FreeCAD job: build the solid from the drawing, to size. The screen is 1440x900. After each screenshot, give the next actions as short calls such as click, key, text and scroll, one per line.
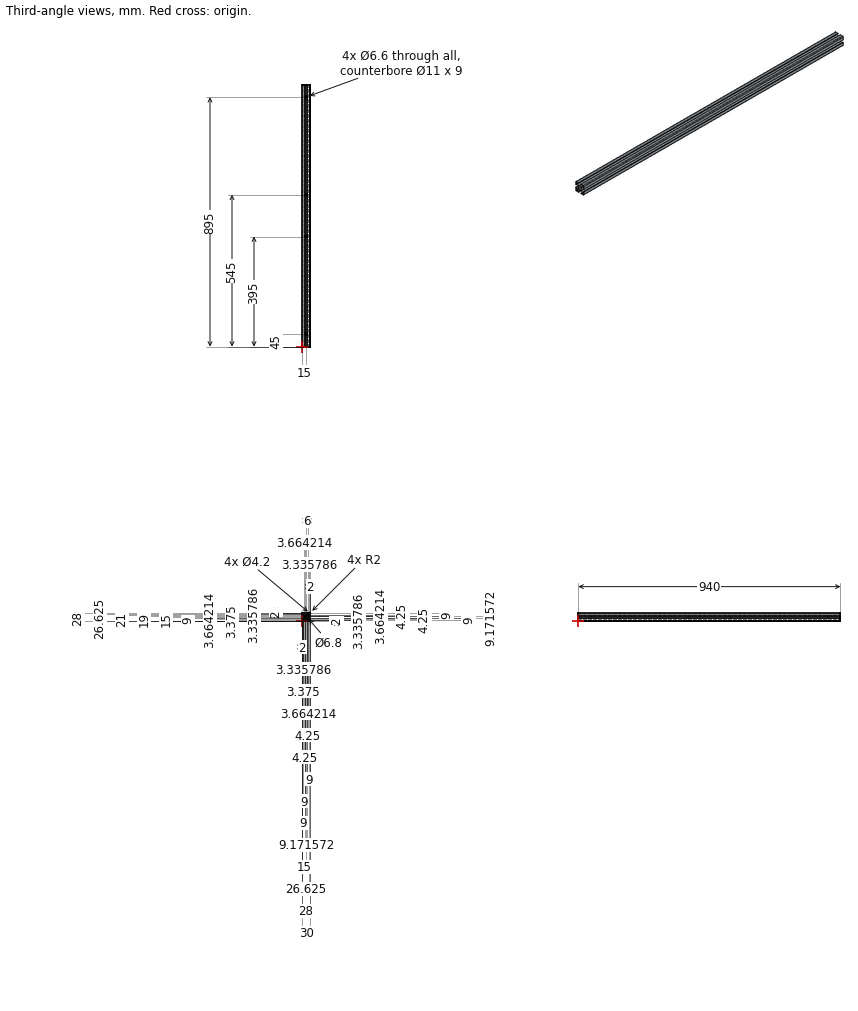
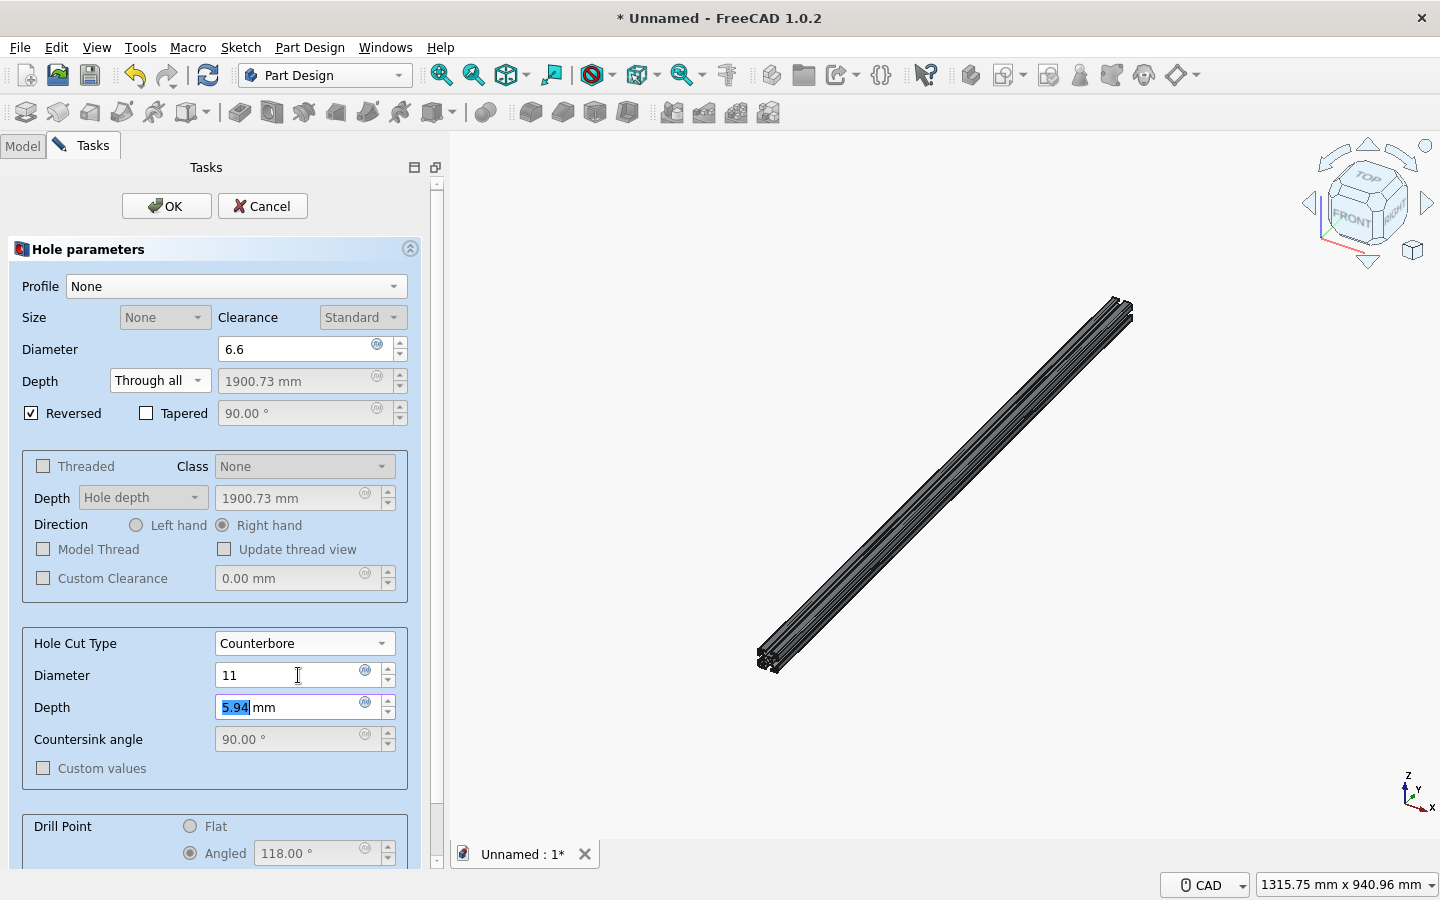
text(9)
key(Tab)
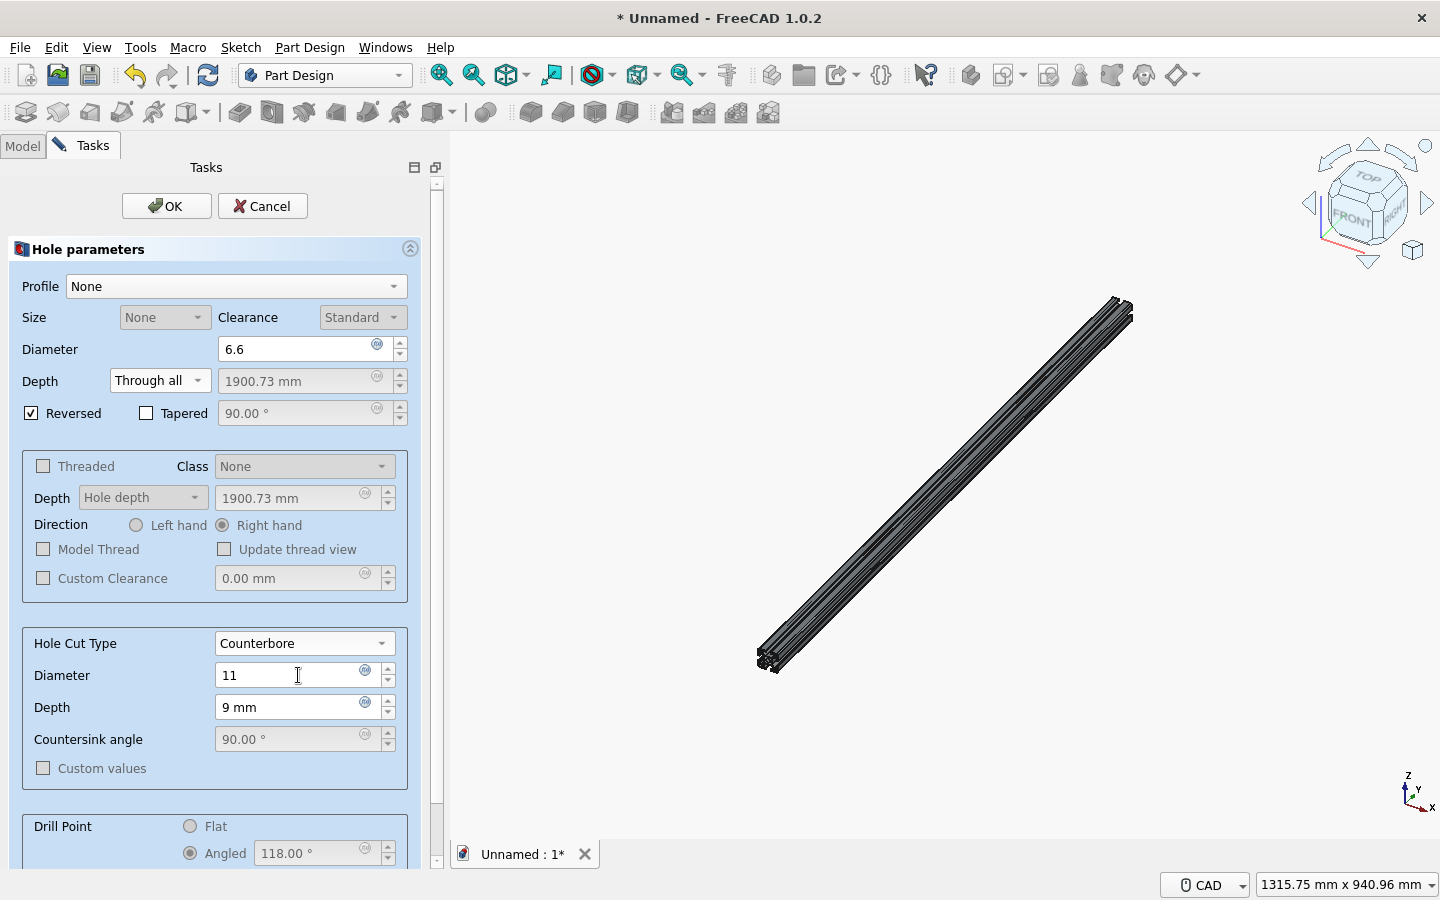
click(167, 206)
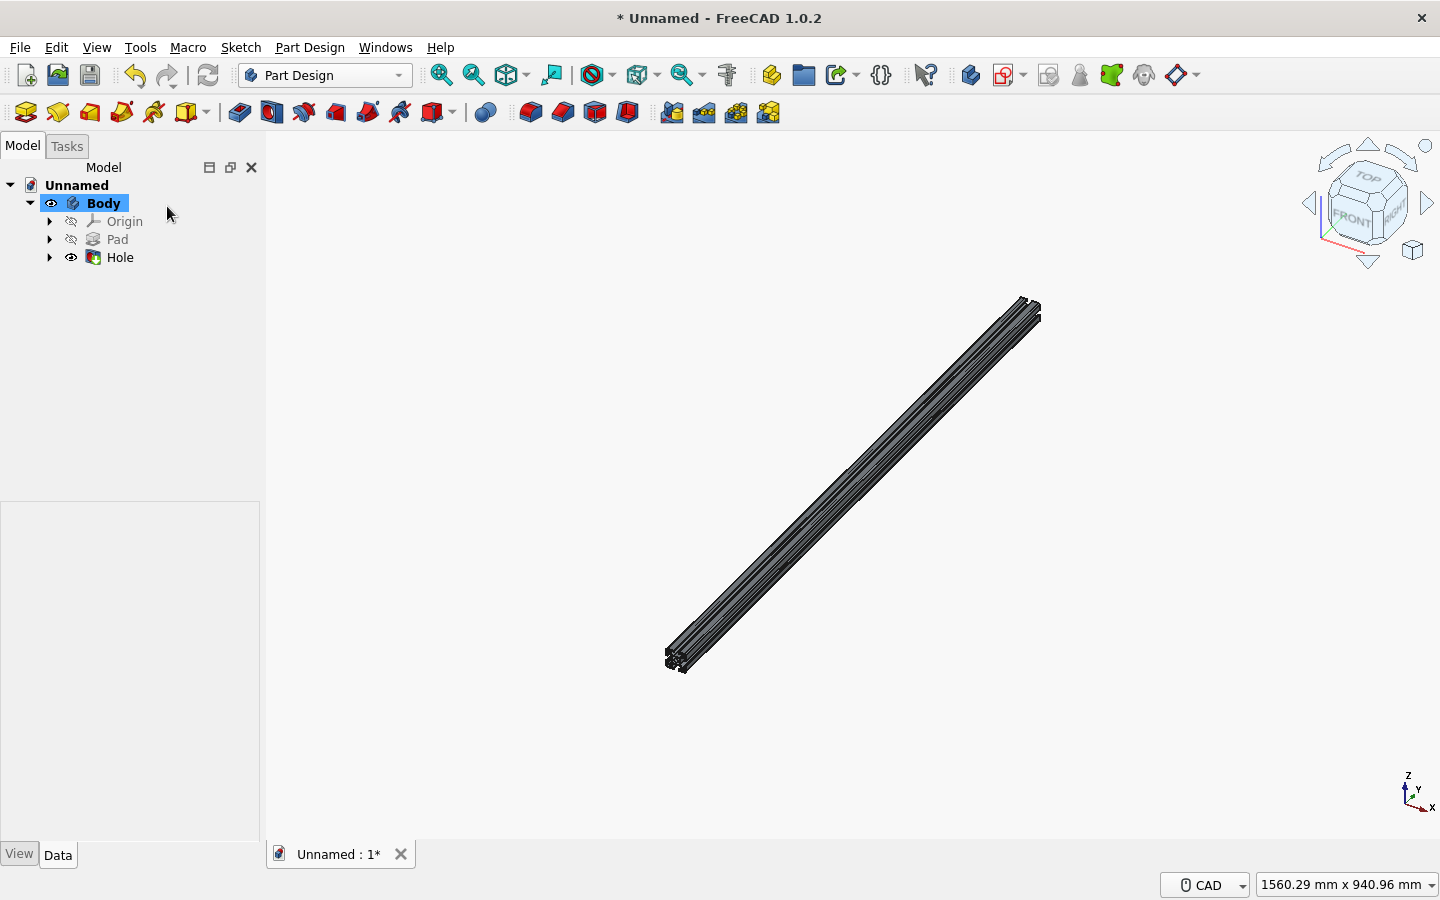
key(0)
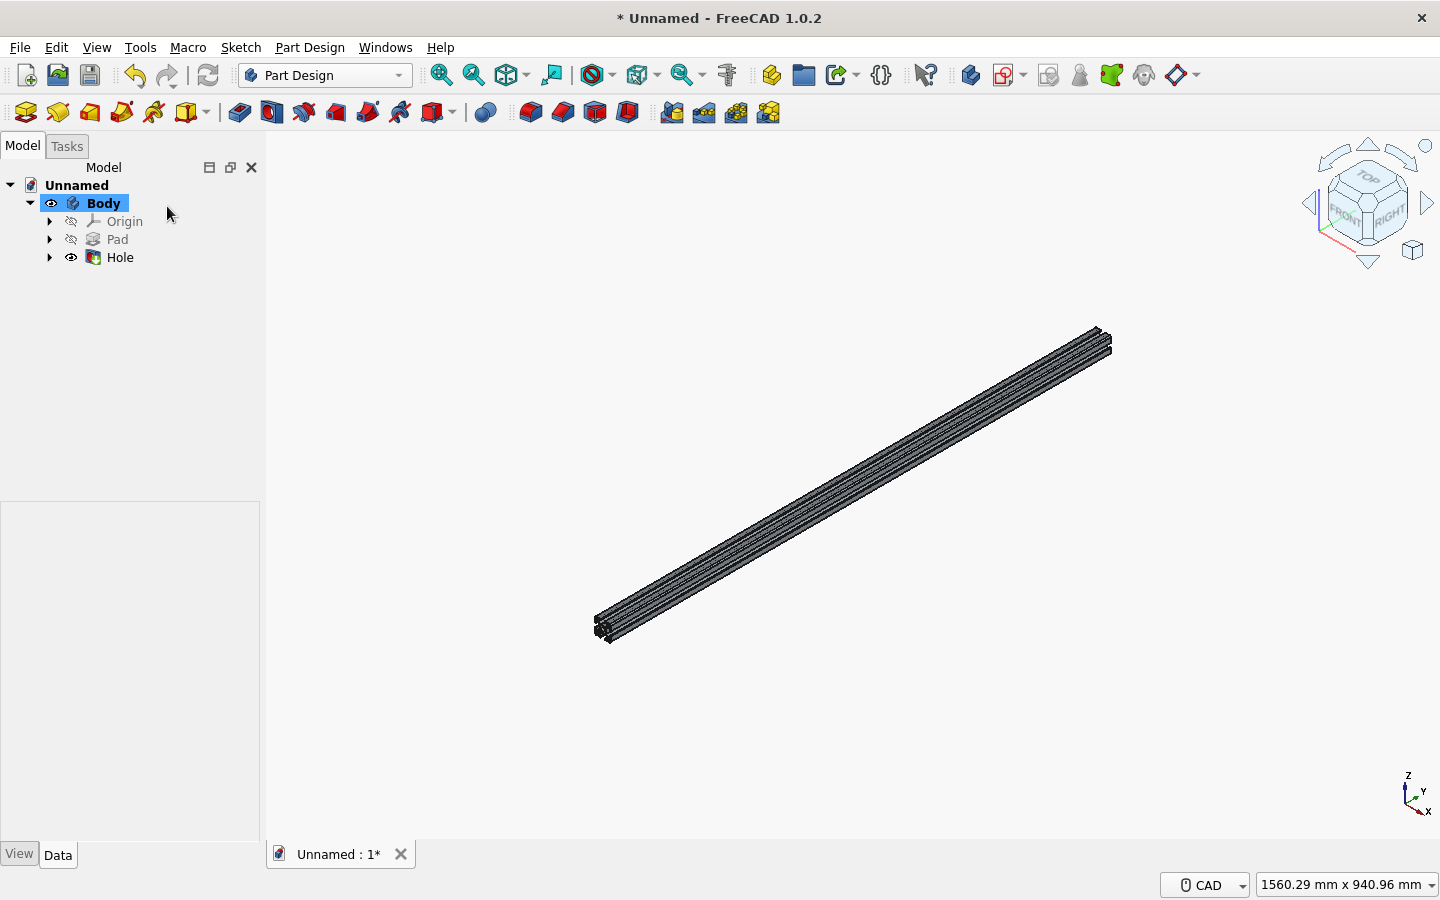
click(442, 76)